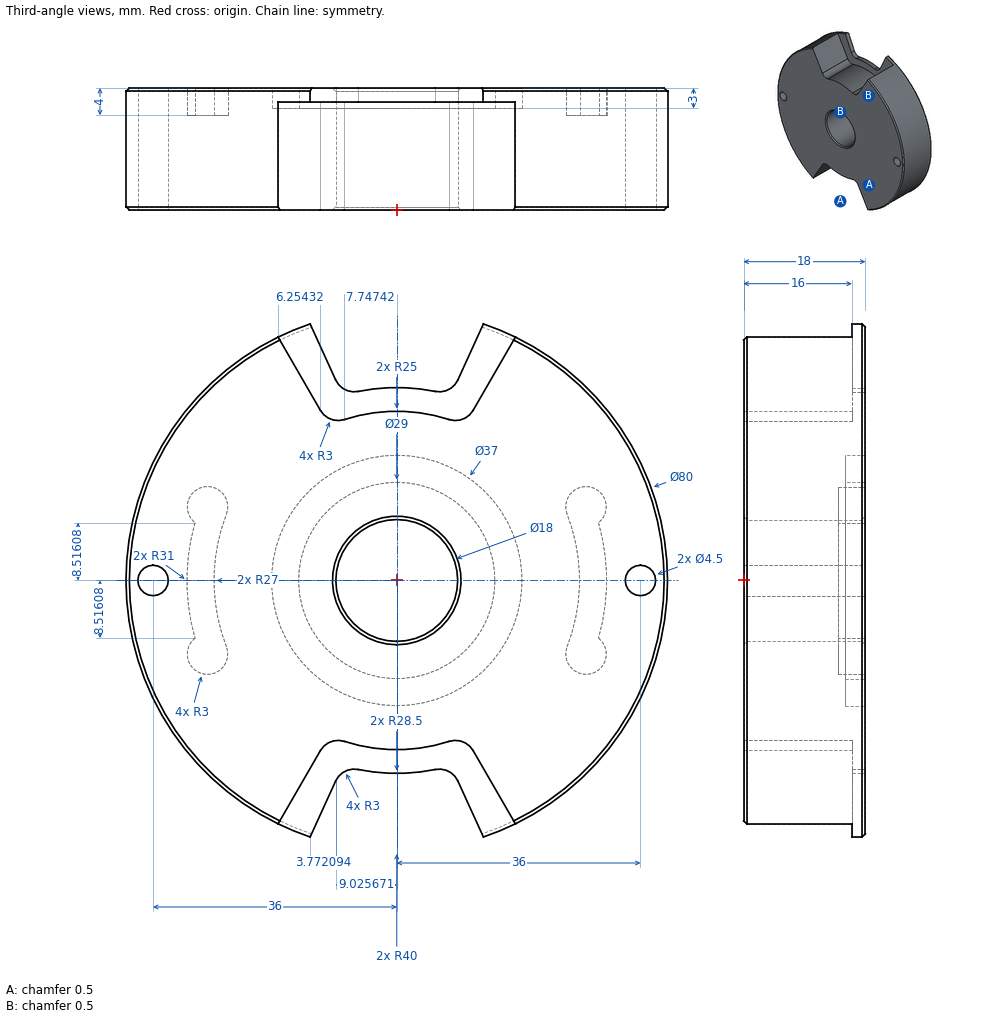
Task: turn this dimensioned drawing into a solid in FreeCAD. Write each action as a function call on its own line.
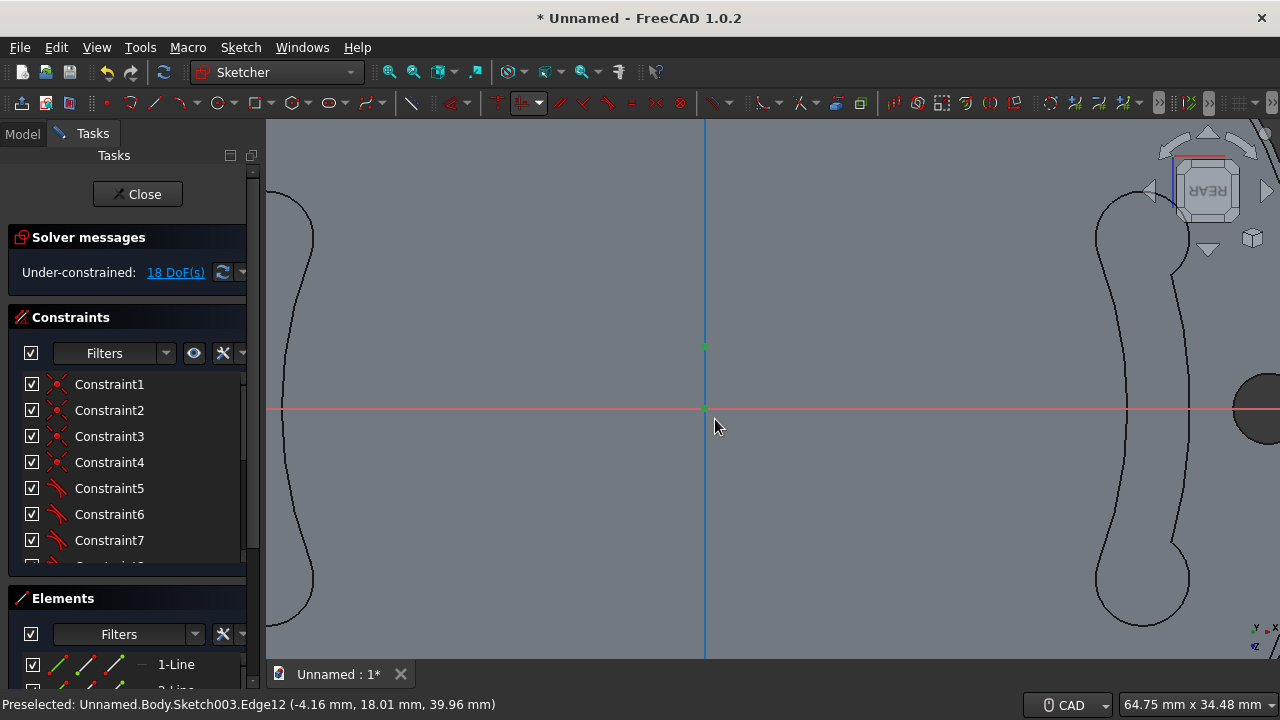
click(498, 104)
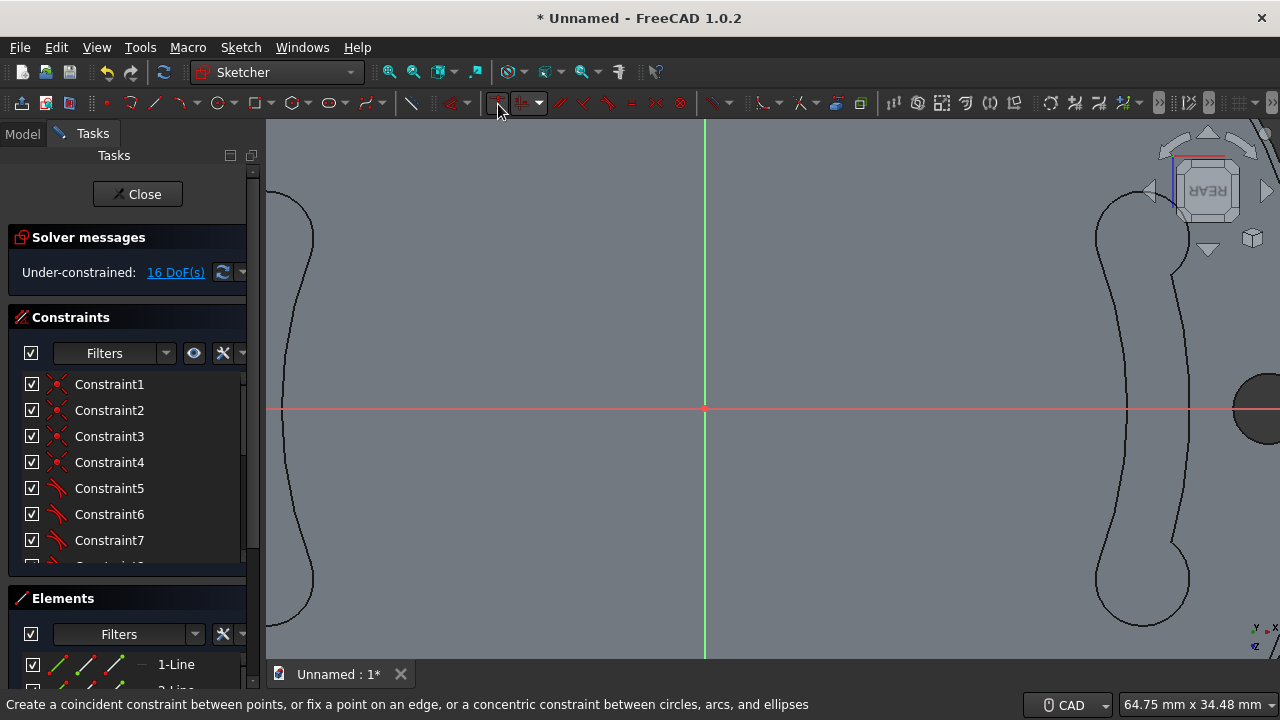
scroll(704, 380, down, 6)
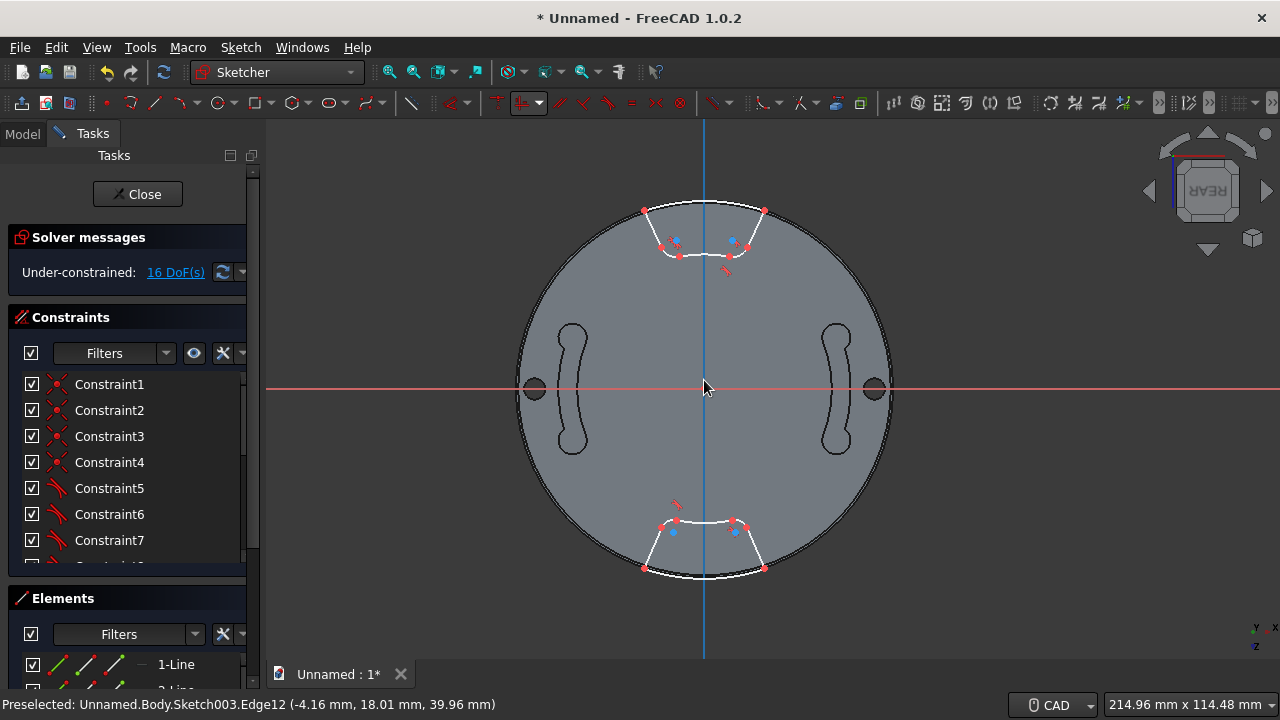
scroll(665, 253, up, 4)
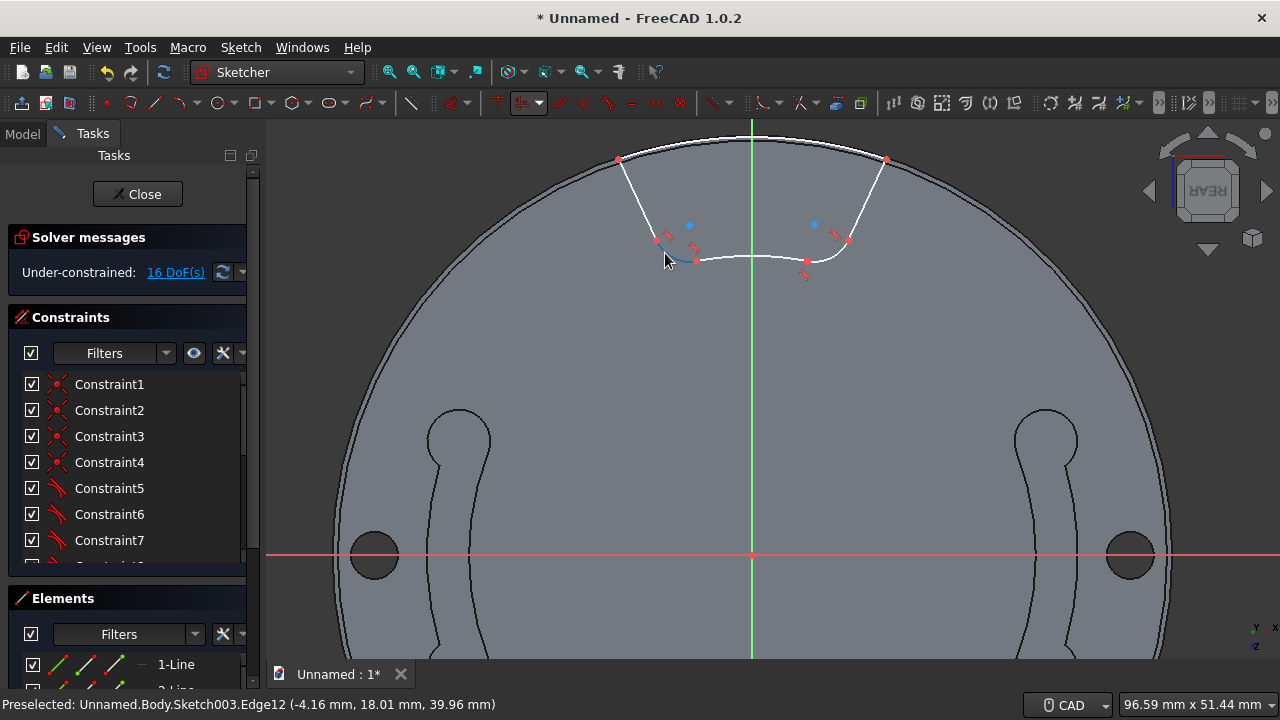
click(665, 252)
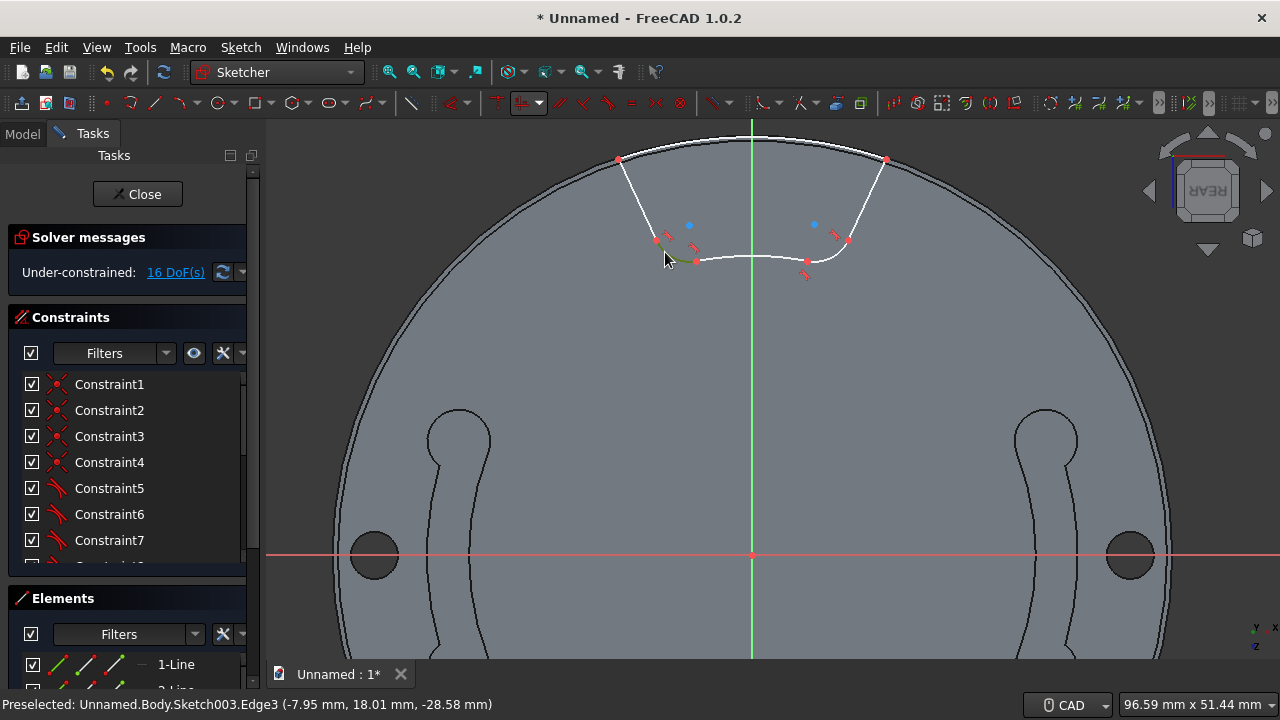
click(822, 261)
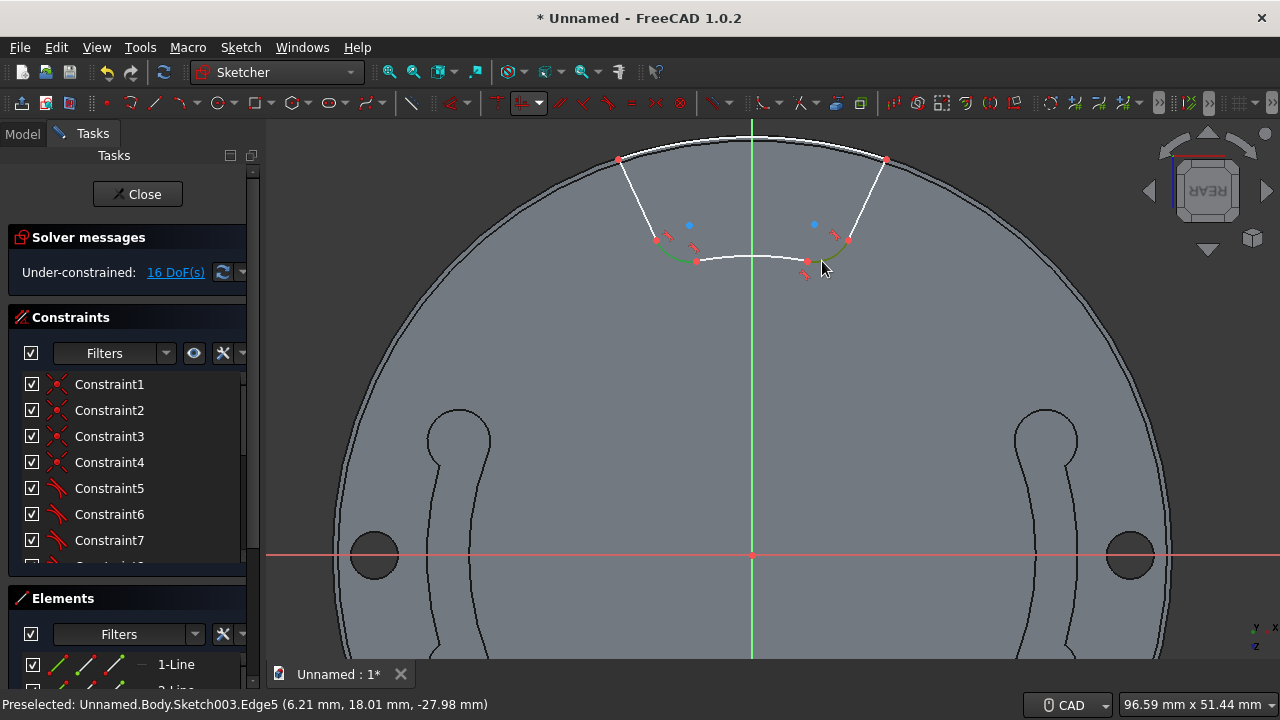
scroll(665, 253, down, 4)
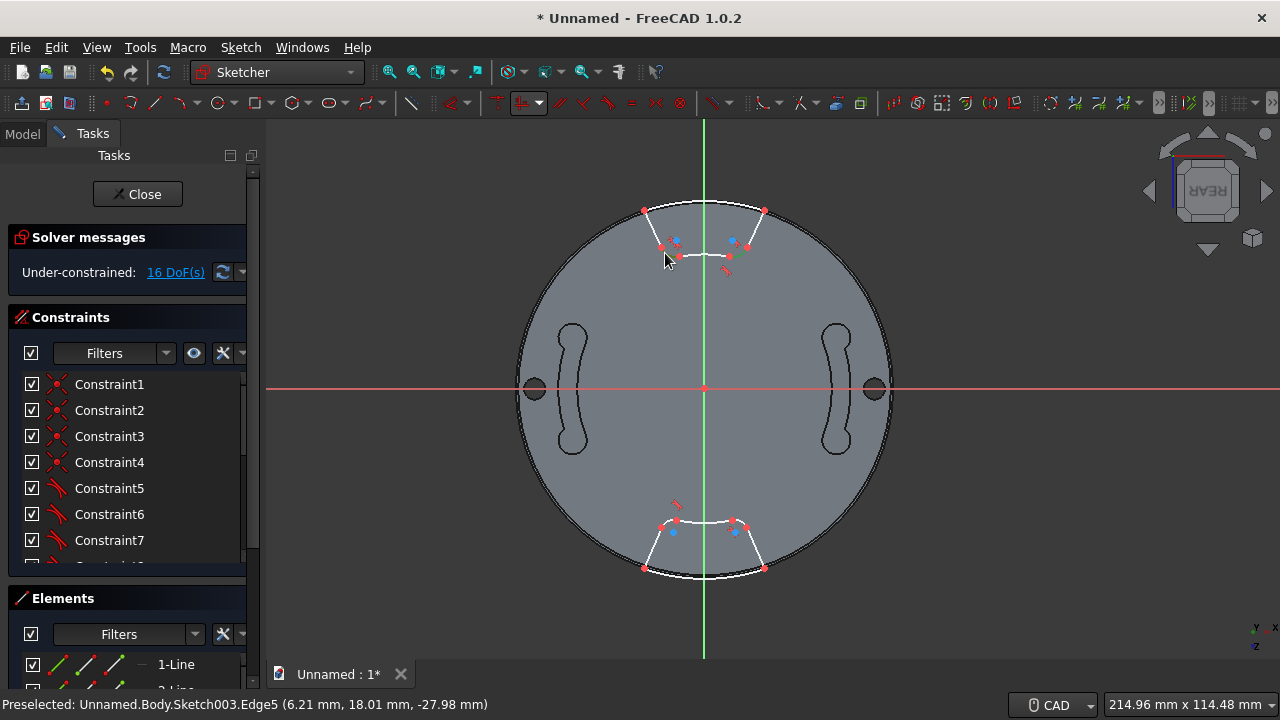
scroll(744, 523, up, 5)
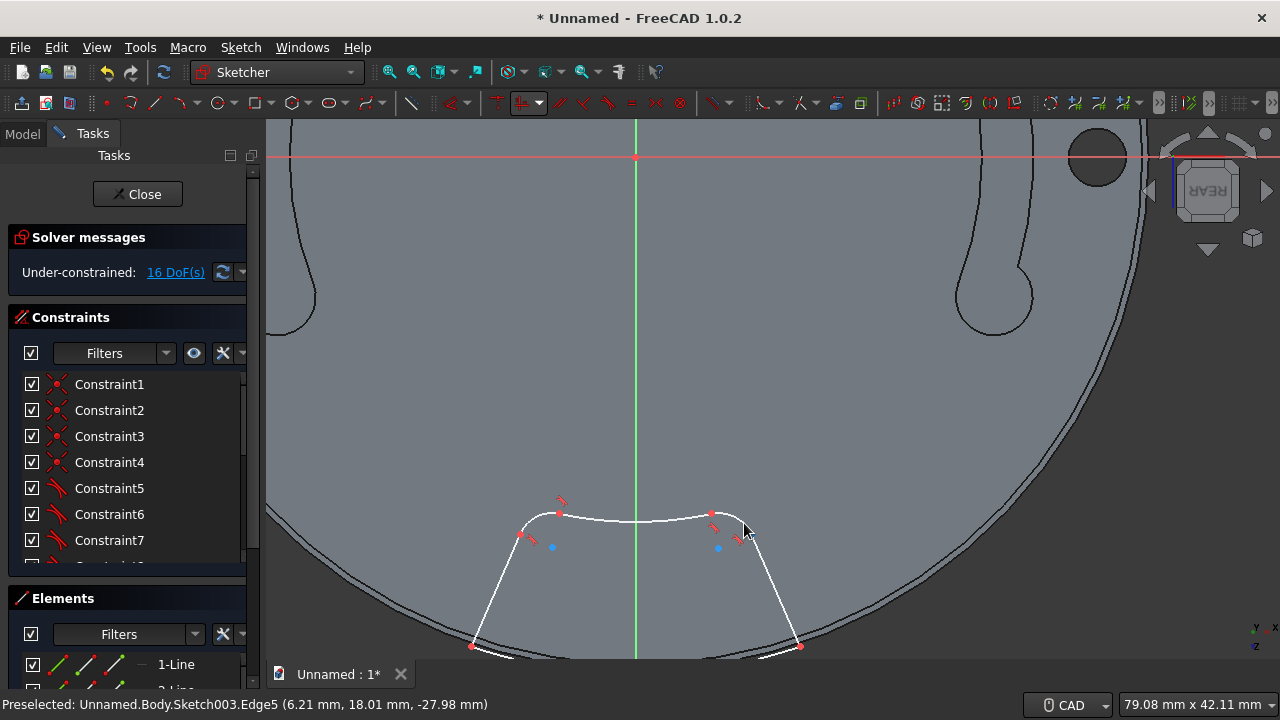
click(743, 523)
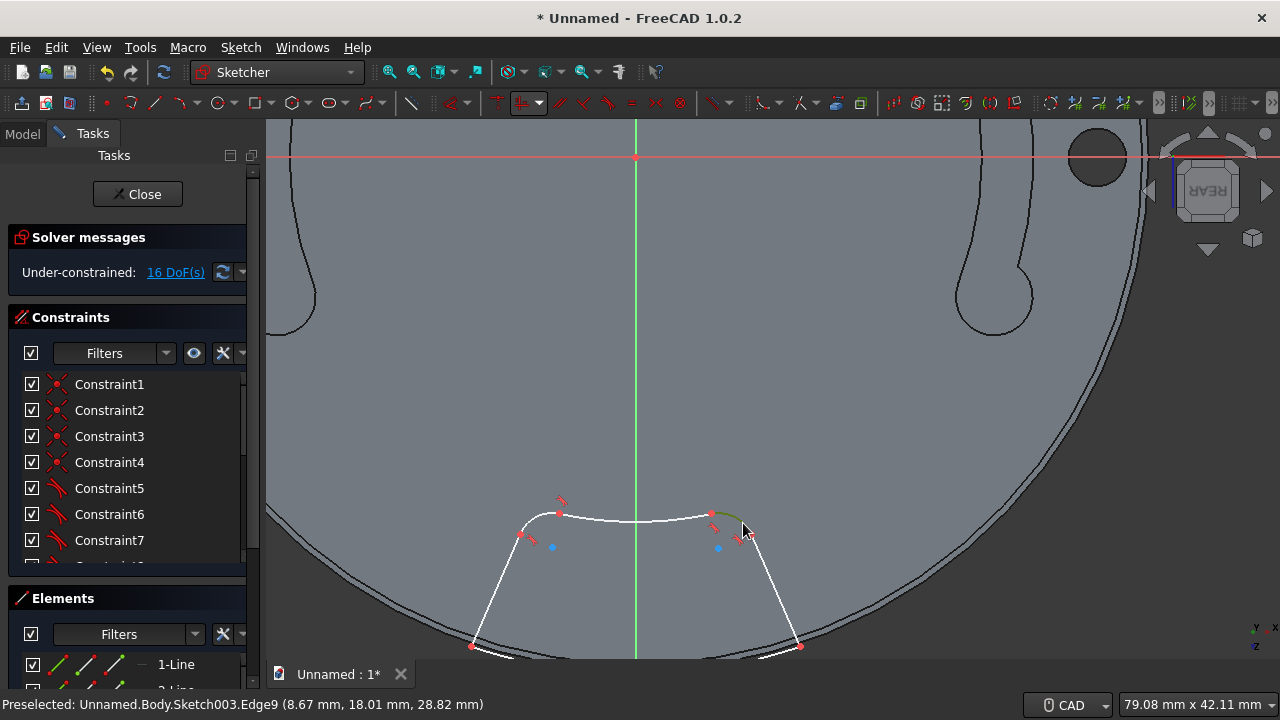
click(545, 514)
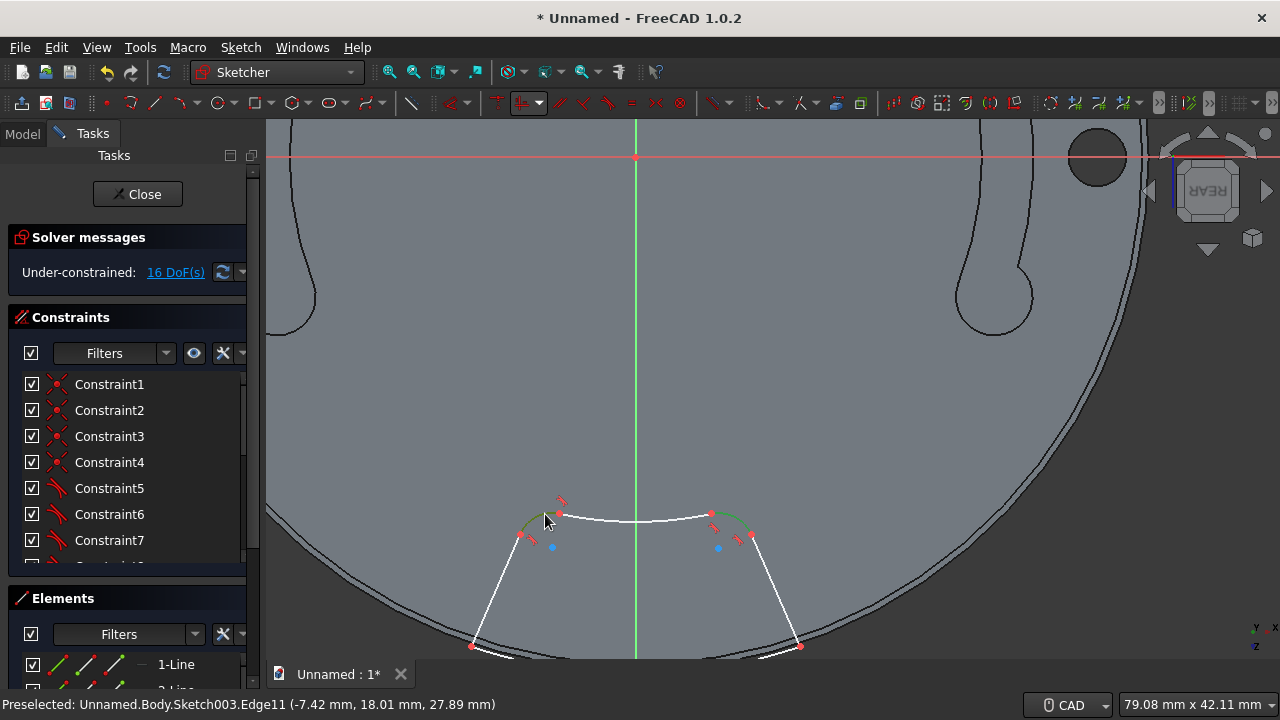
click(632, 104)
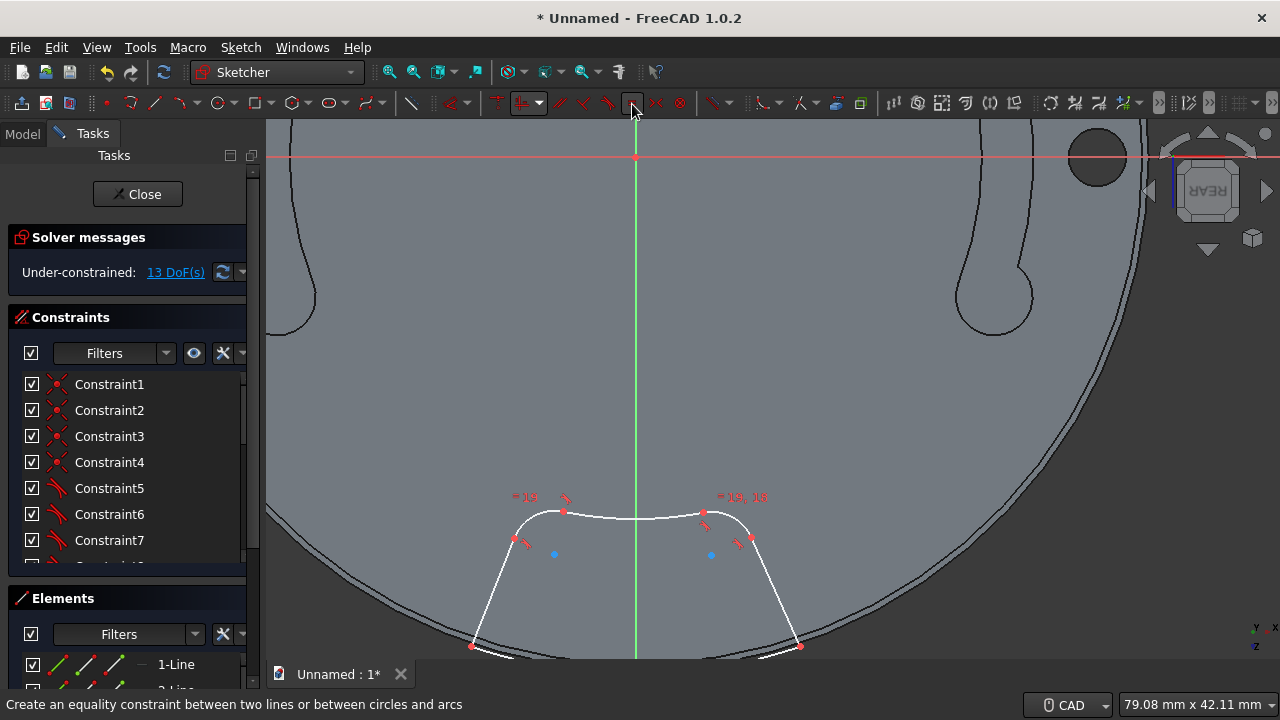
scroll(744, 524, down, 5)